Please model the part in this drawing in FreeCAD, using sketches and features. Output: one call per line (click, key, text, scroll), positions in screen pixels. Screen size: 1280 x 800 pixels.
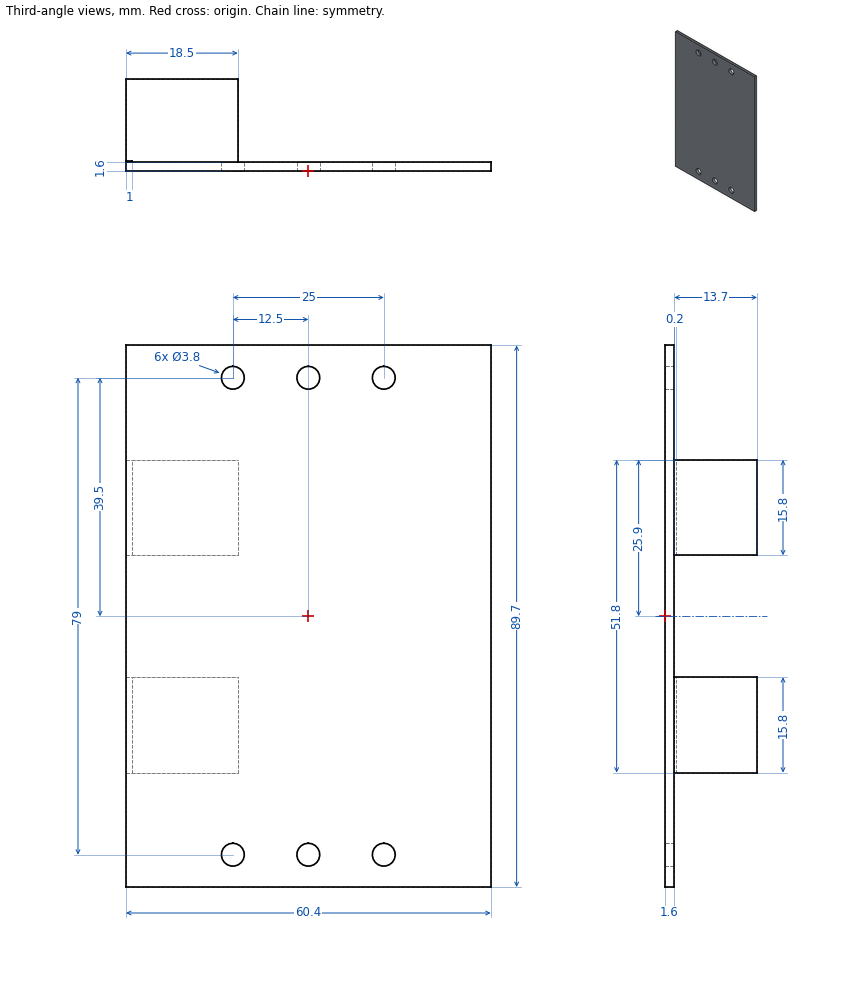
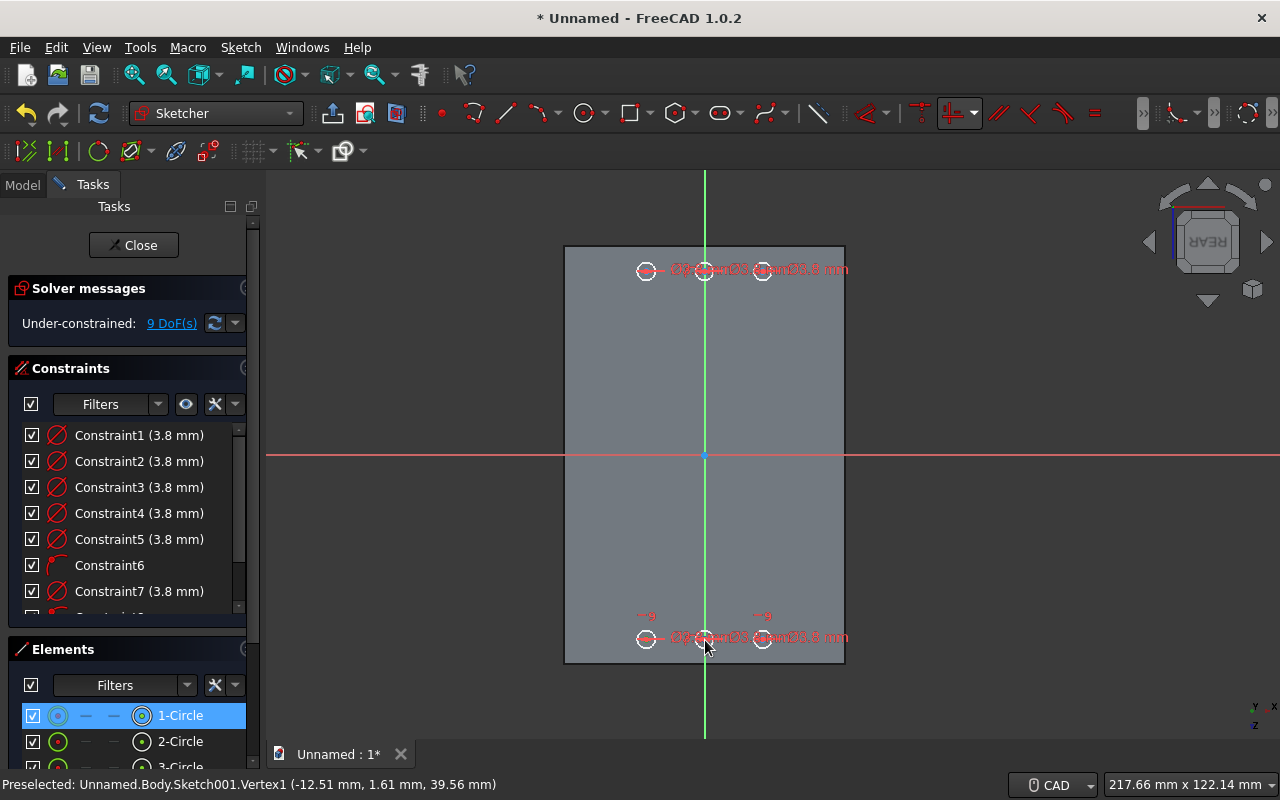
click(646, 271)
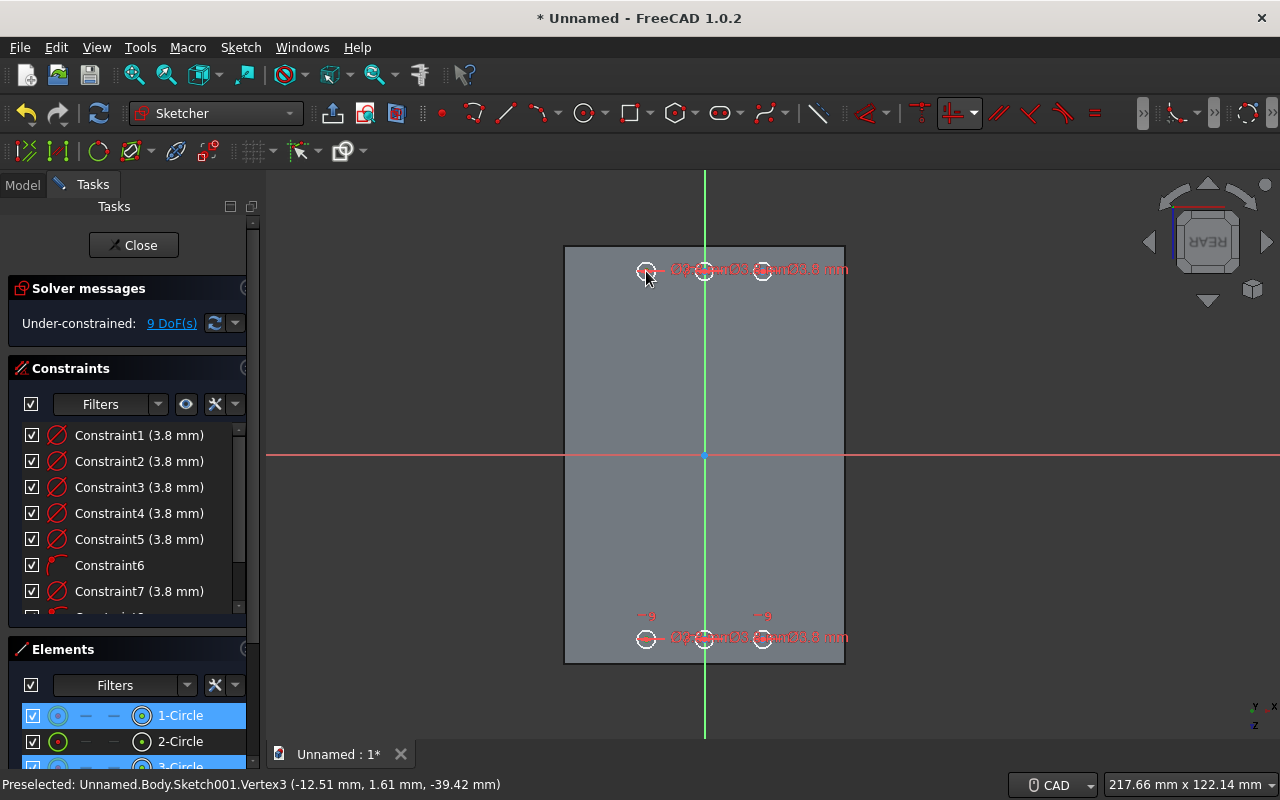
key(v)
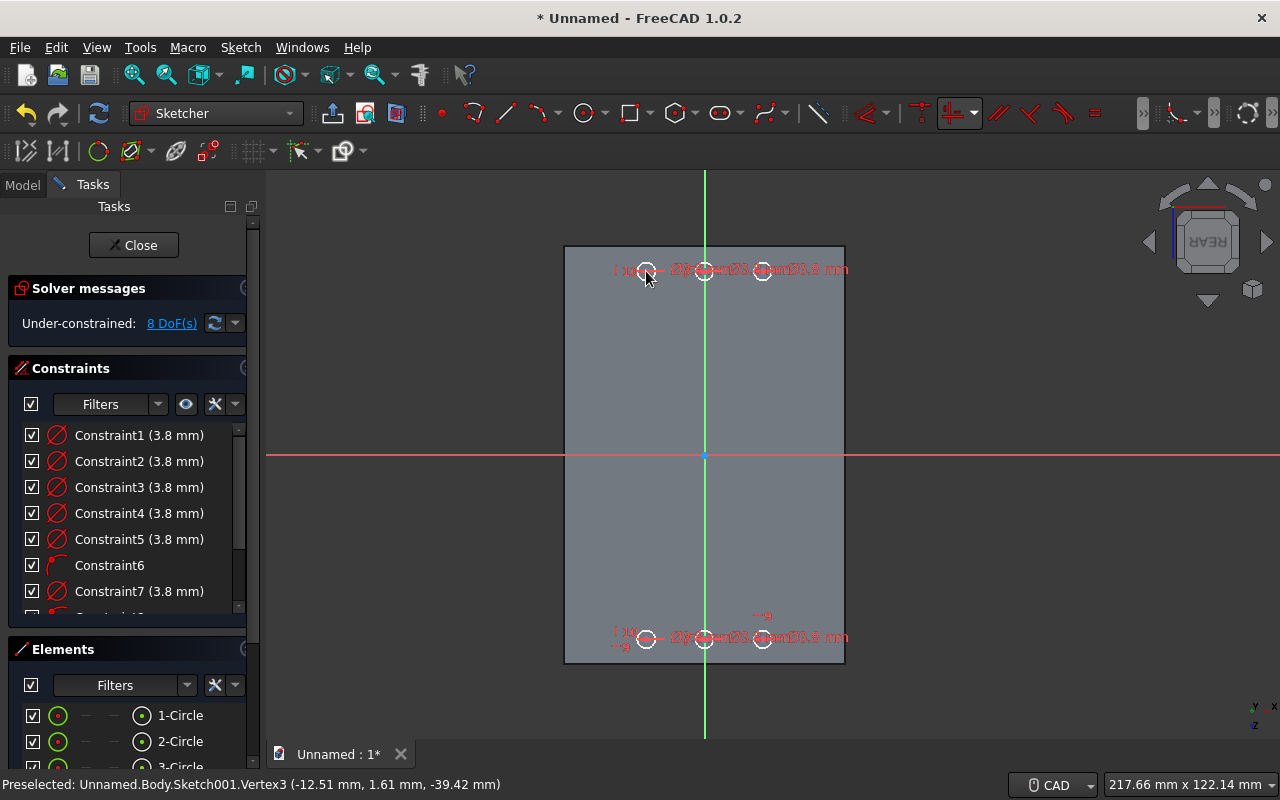
click(763, 639)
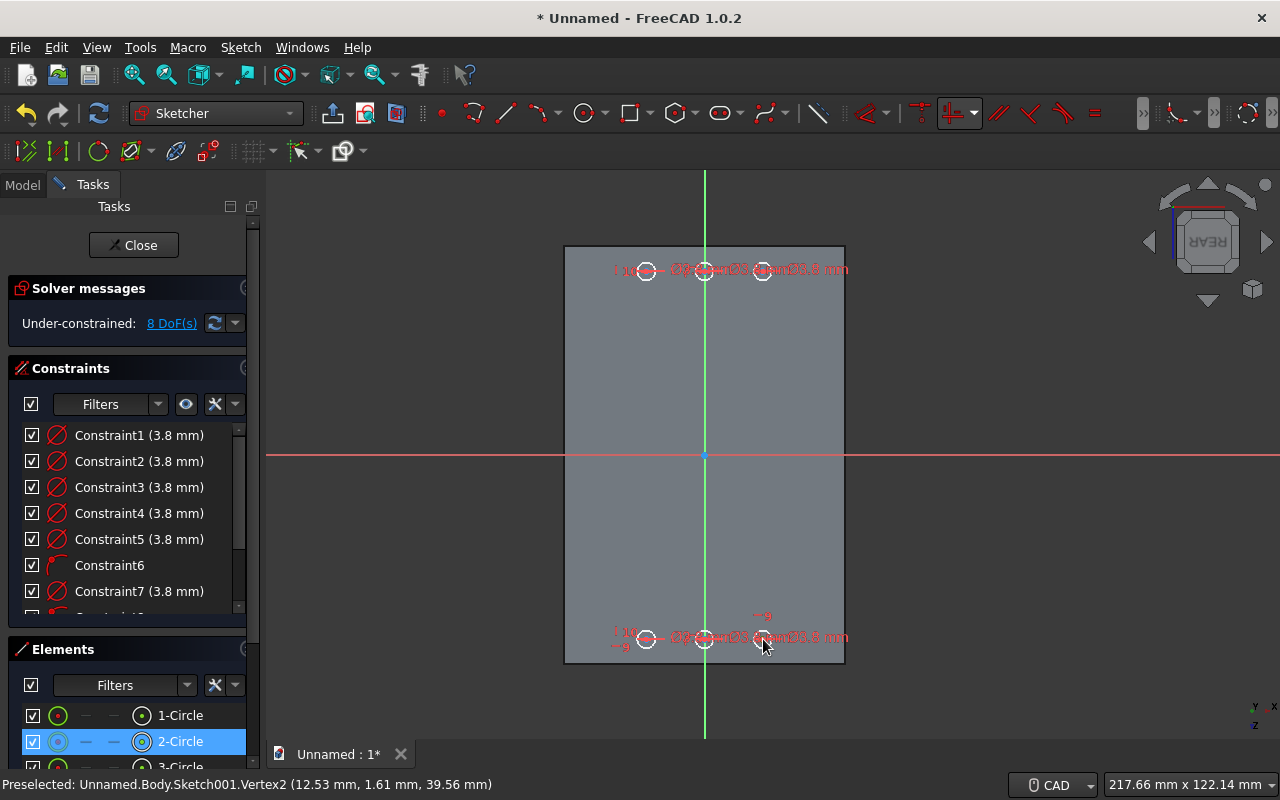
click(763, 271)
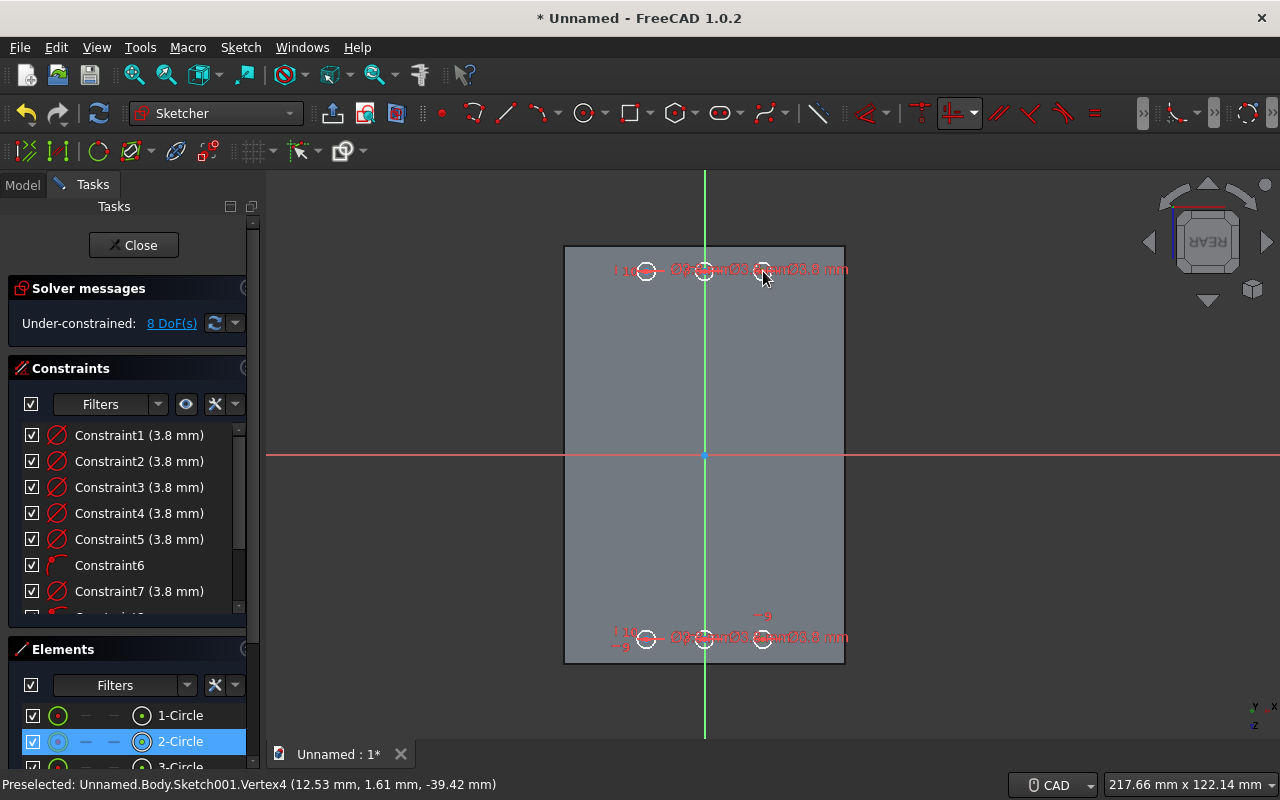
key(v)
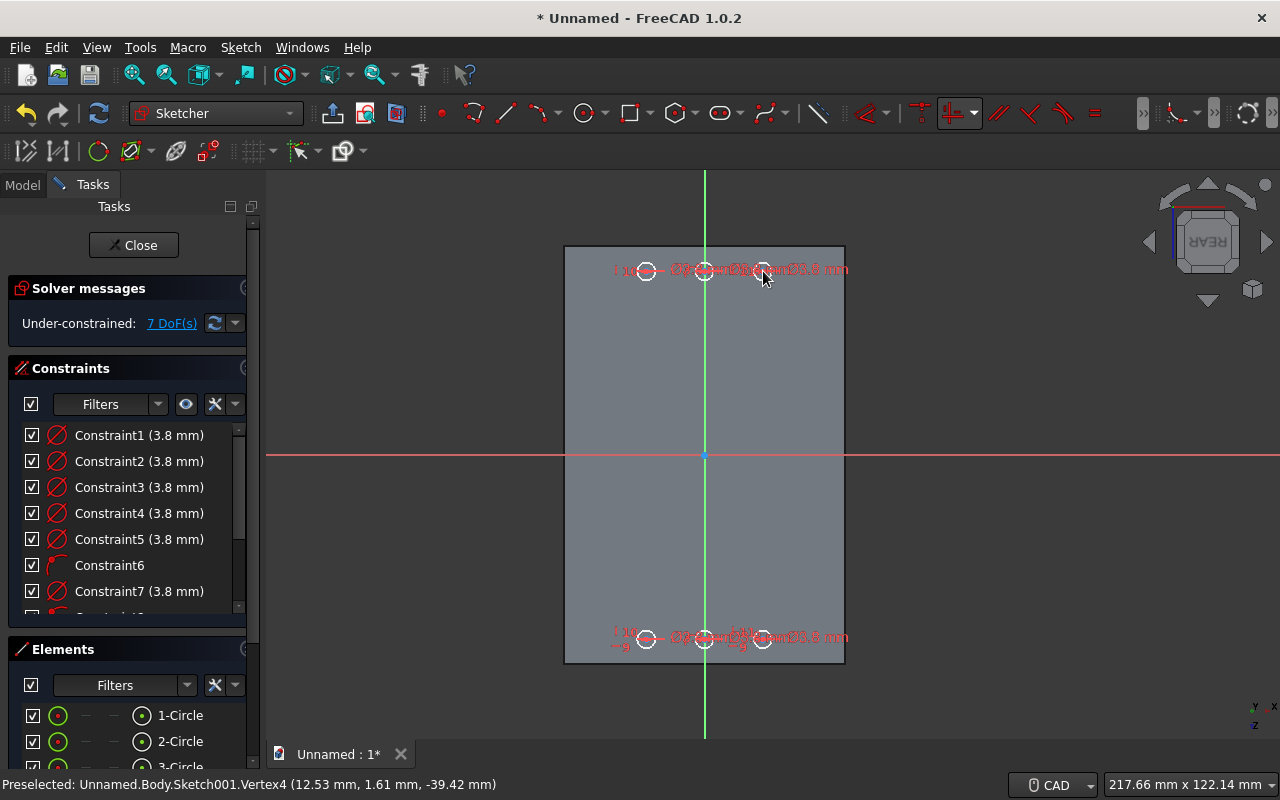
click(646, 271)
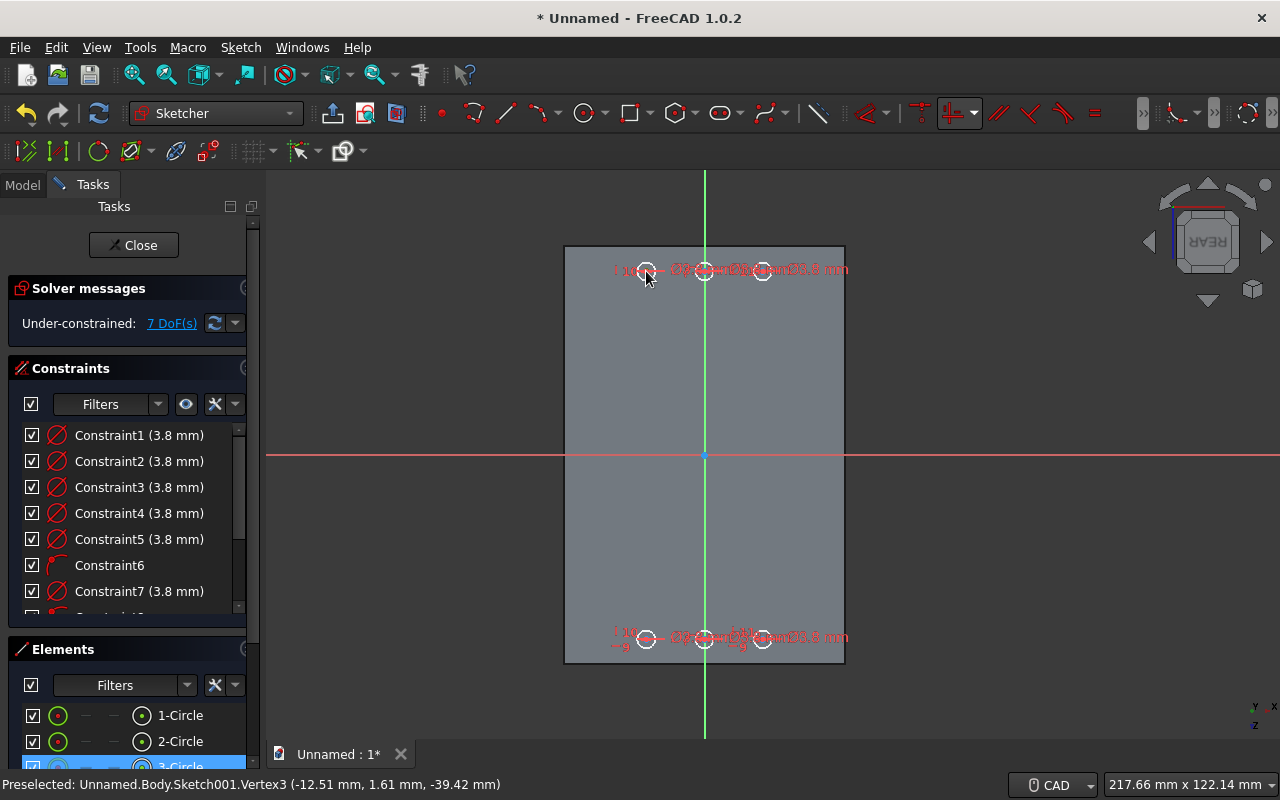
click(763, 271)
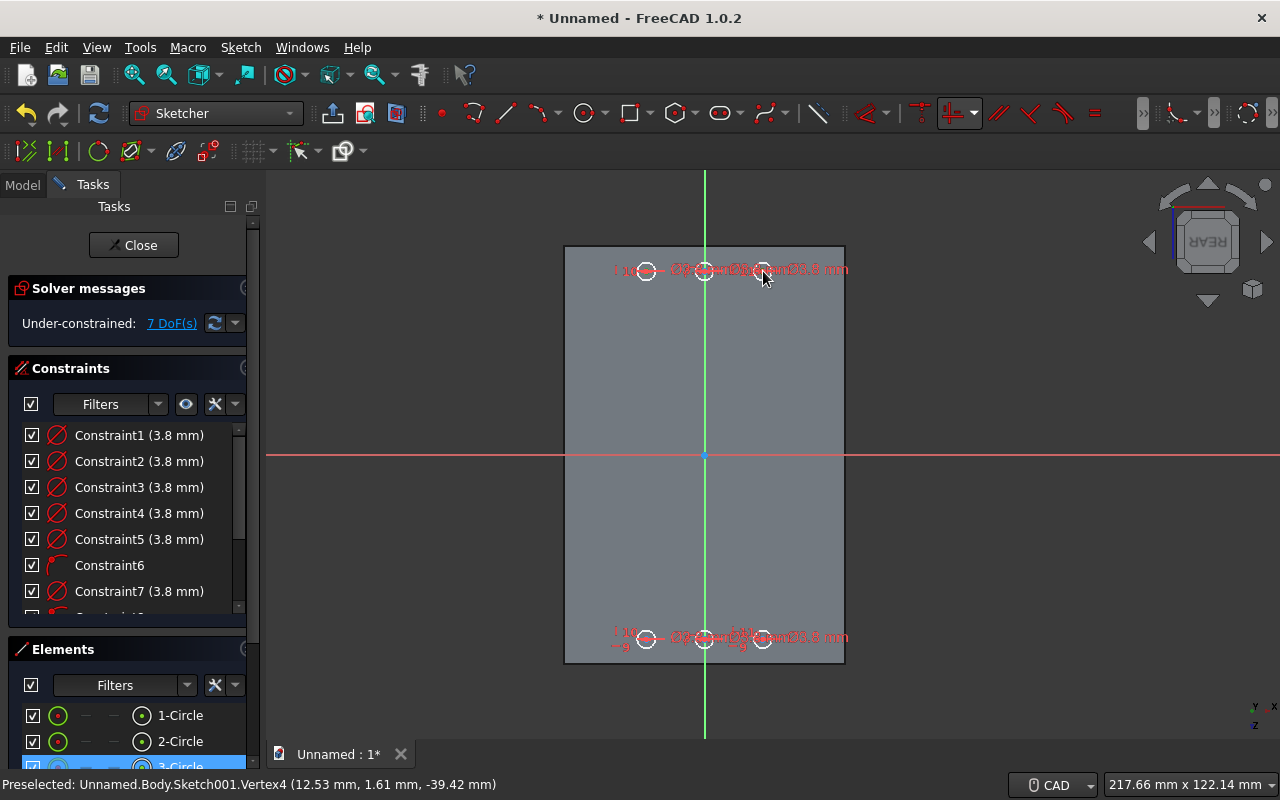
click(976, 114)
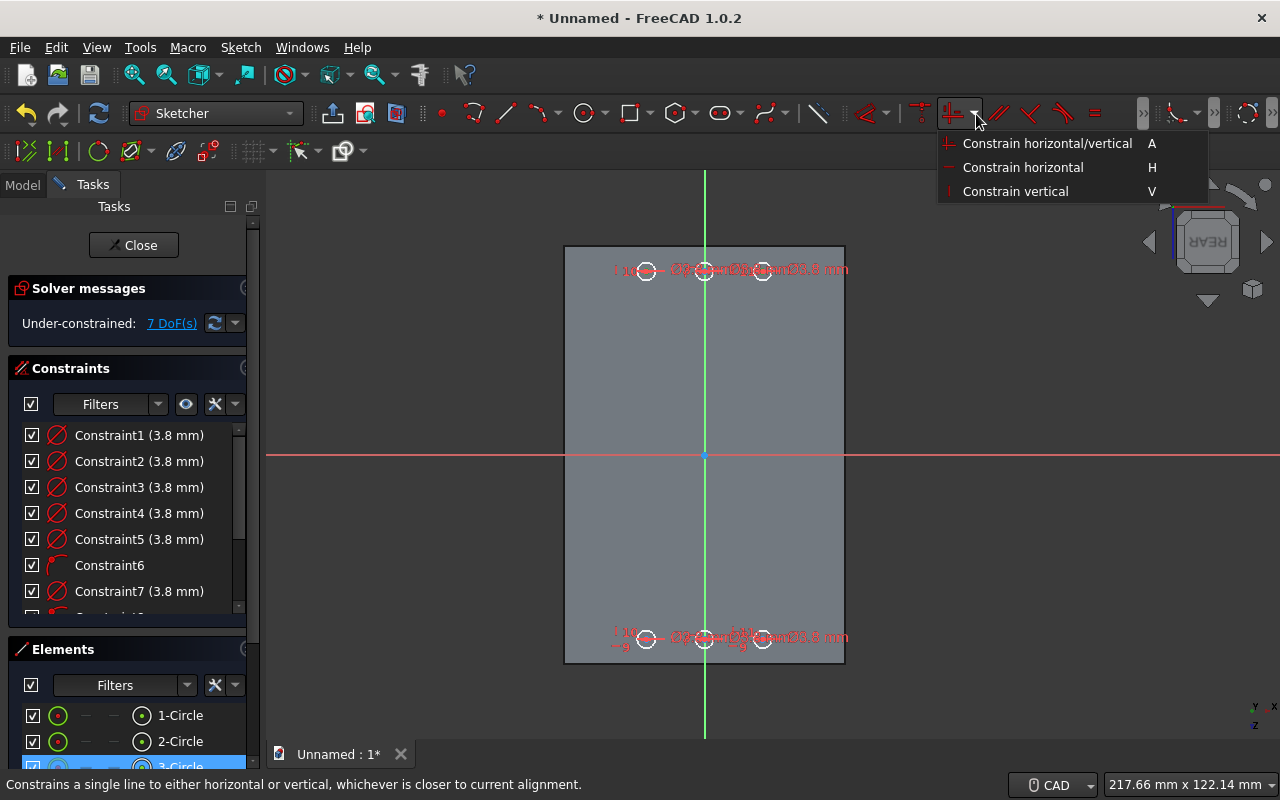
click(1073, 167)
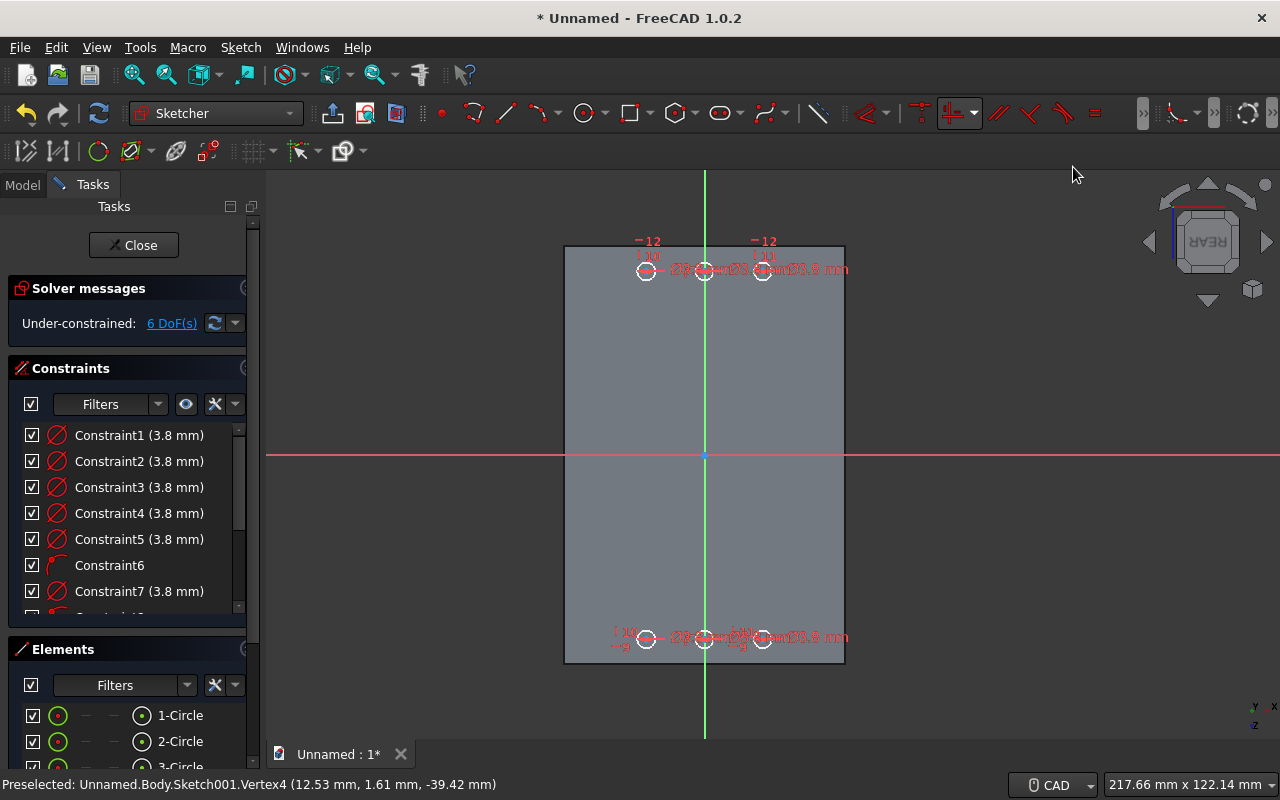
click(646, 271)